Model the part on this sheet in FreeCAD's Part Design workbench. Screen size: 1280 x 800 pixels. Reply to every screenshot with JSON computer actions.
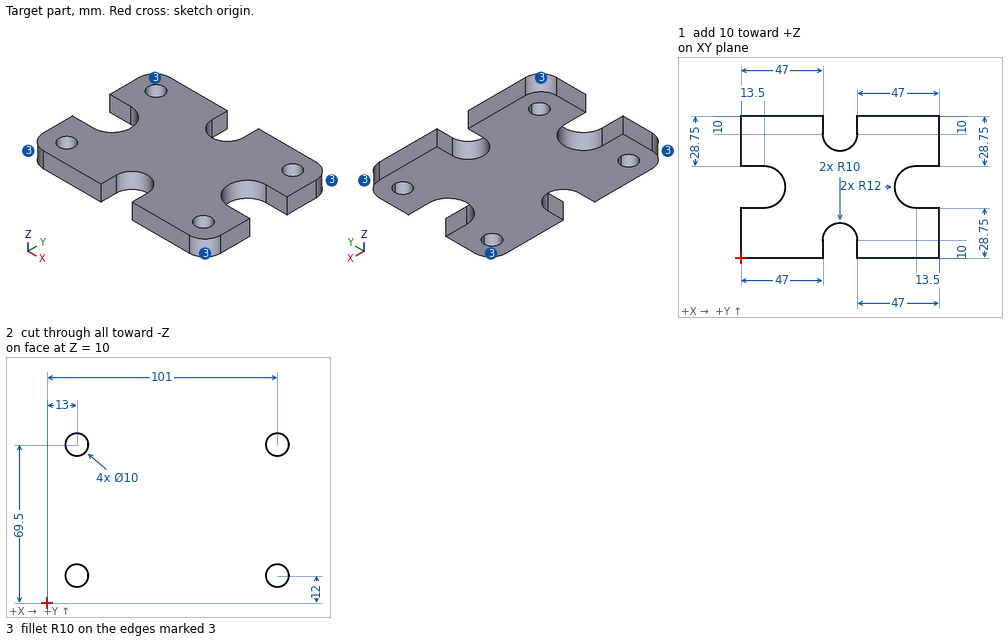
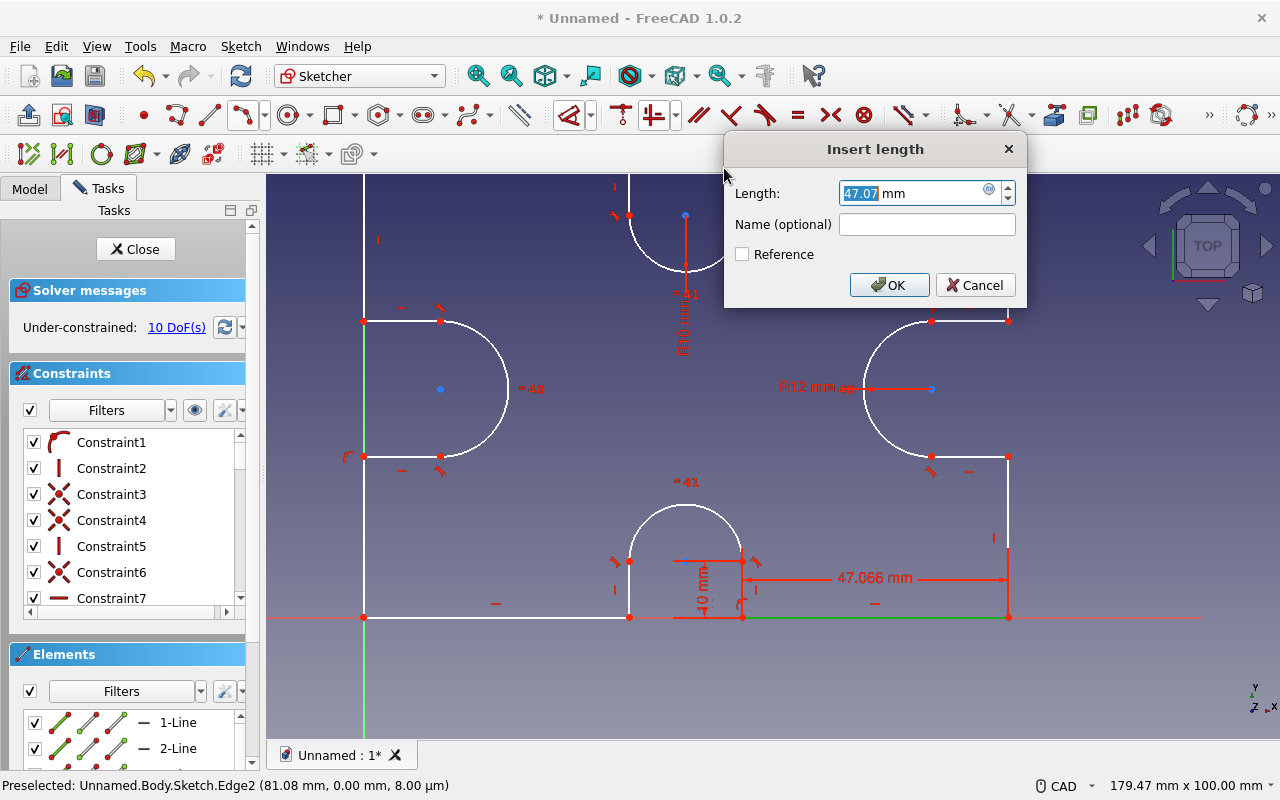
{"action": "type", "text": "47"}
{"action": "key", "text": "Return"}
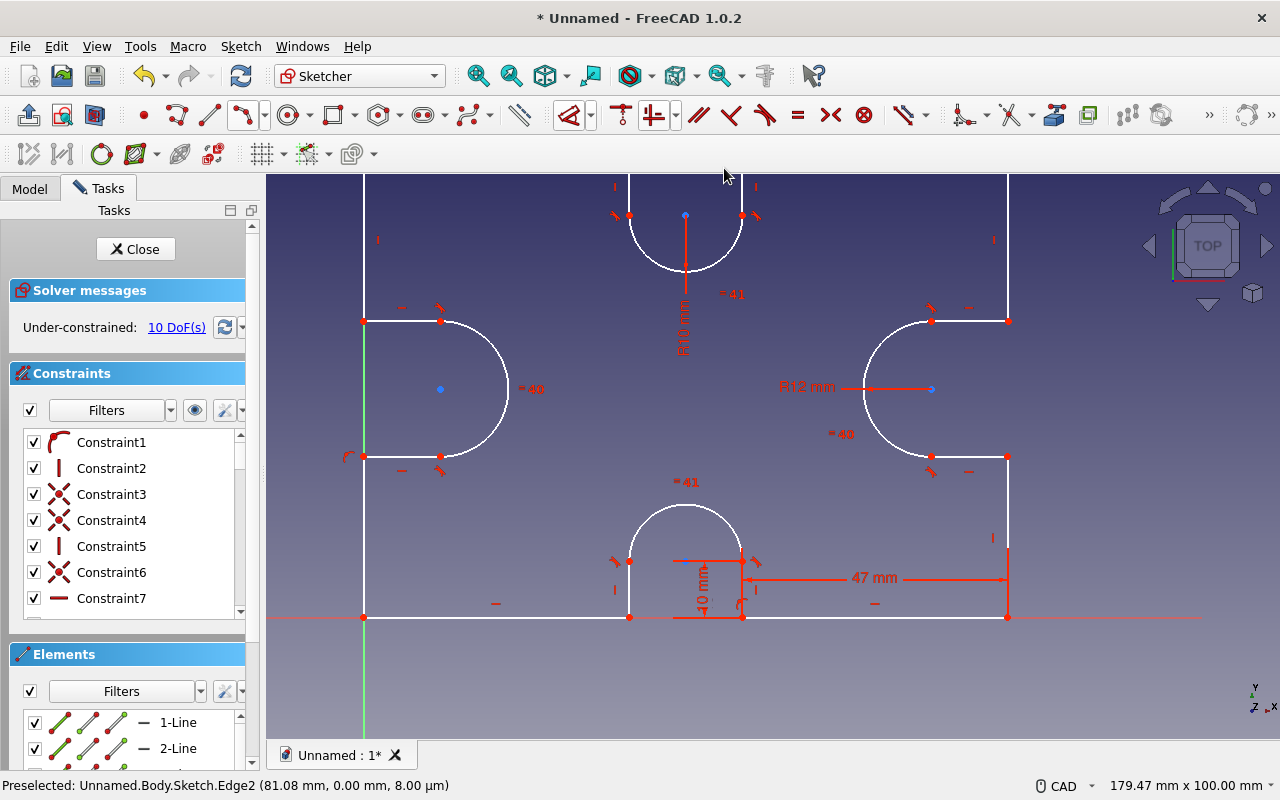
{"action": "scroll", "coordinate": [788, 711], "scroll_direction": "down", "scroll_amount": 1}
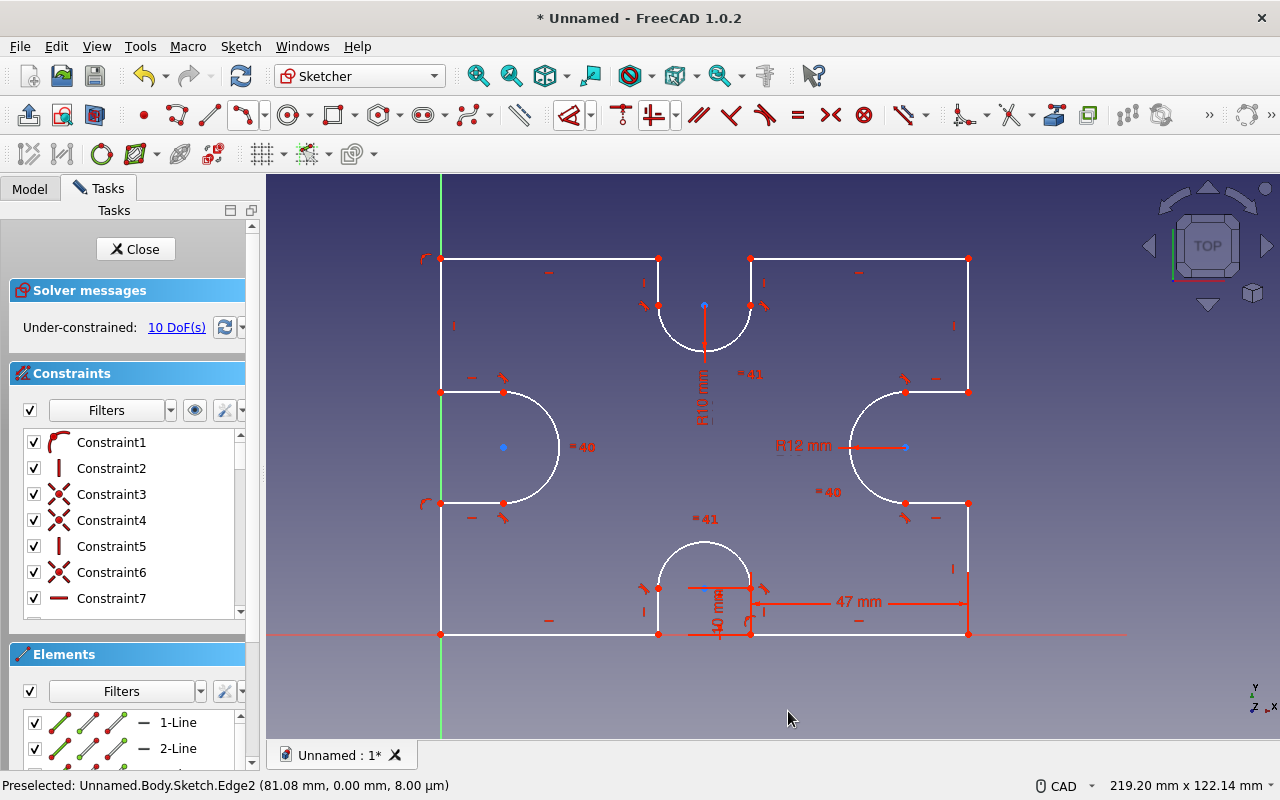
{"action": "left_click", "coordinate": [903, 259]}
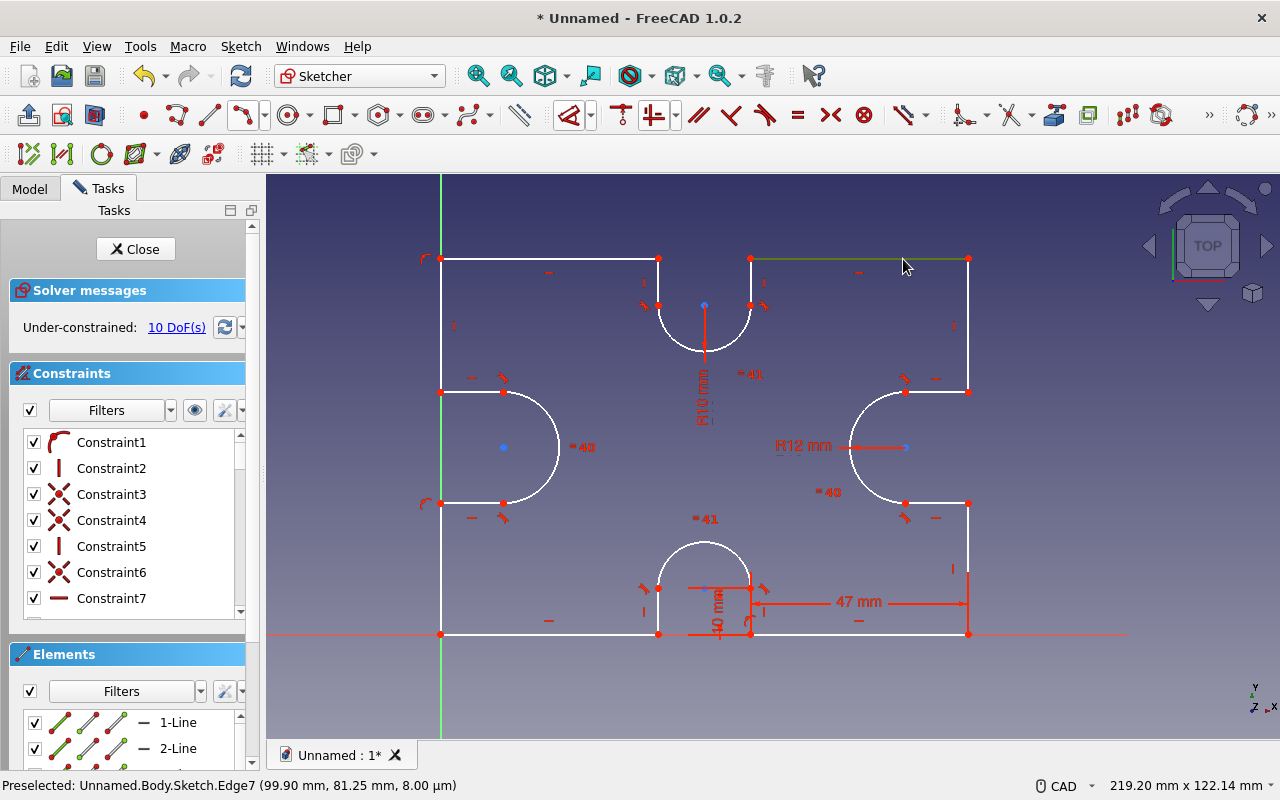
{"action": "left_click", "coordinate": [590, 116]}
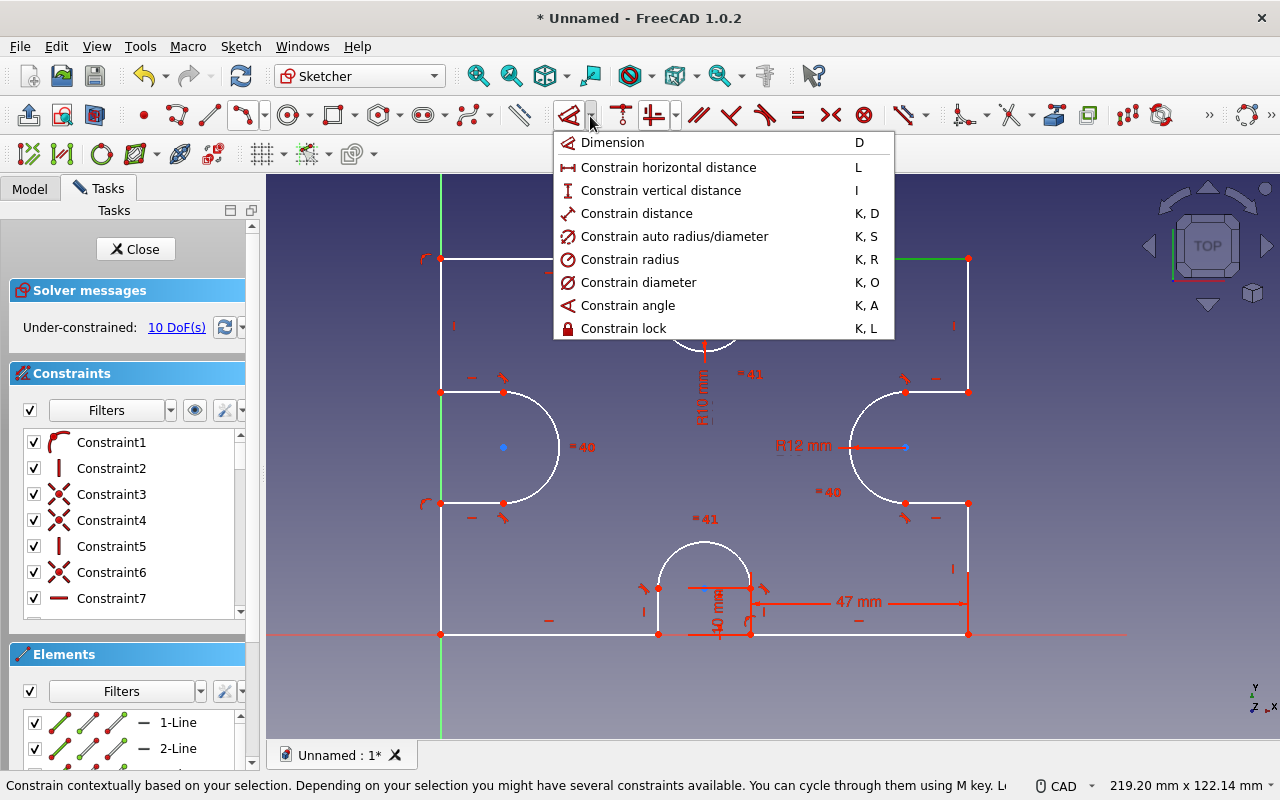
{"action": "left_click", "coordinate": [724, 168]}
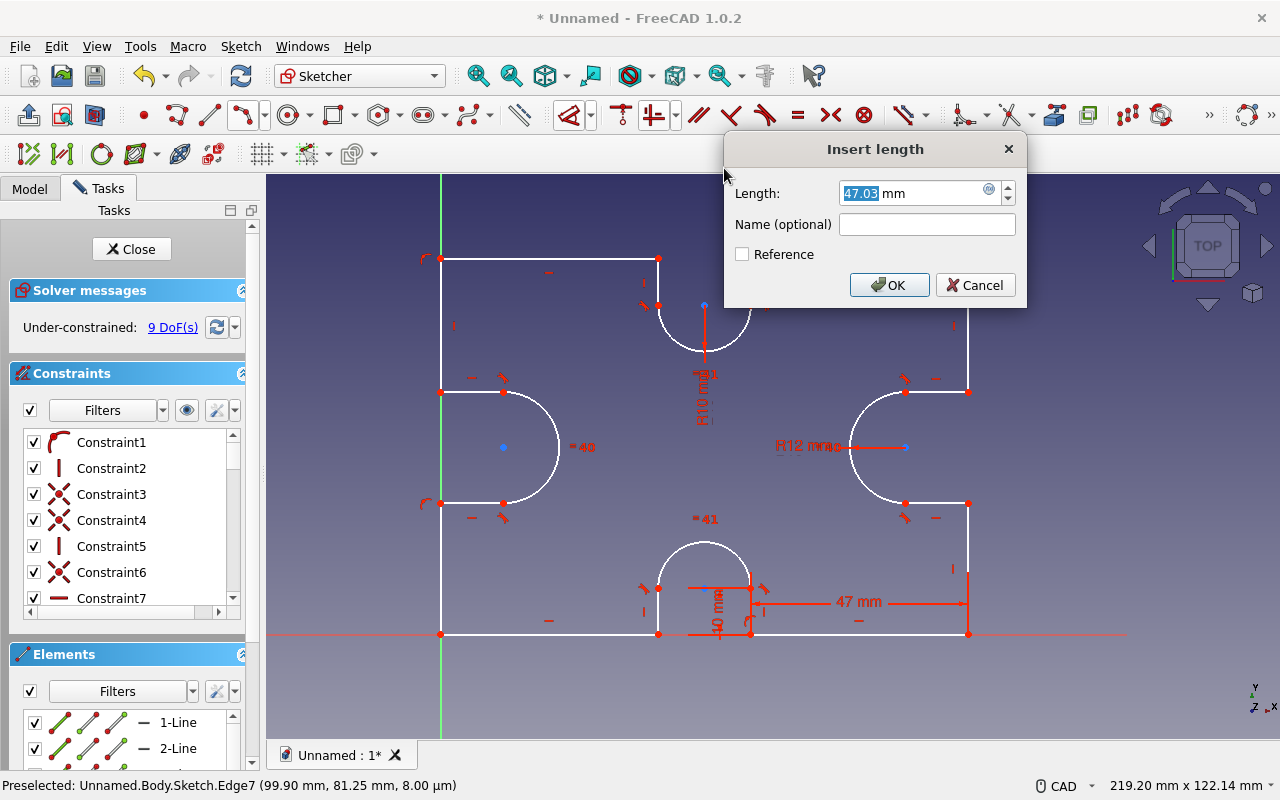
{"action": "type", "text": "47"}
{"action": "key", "text": "Return"}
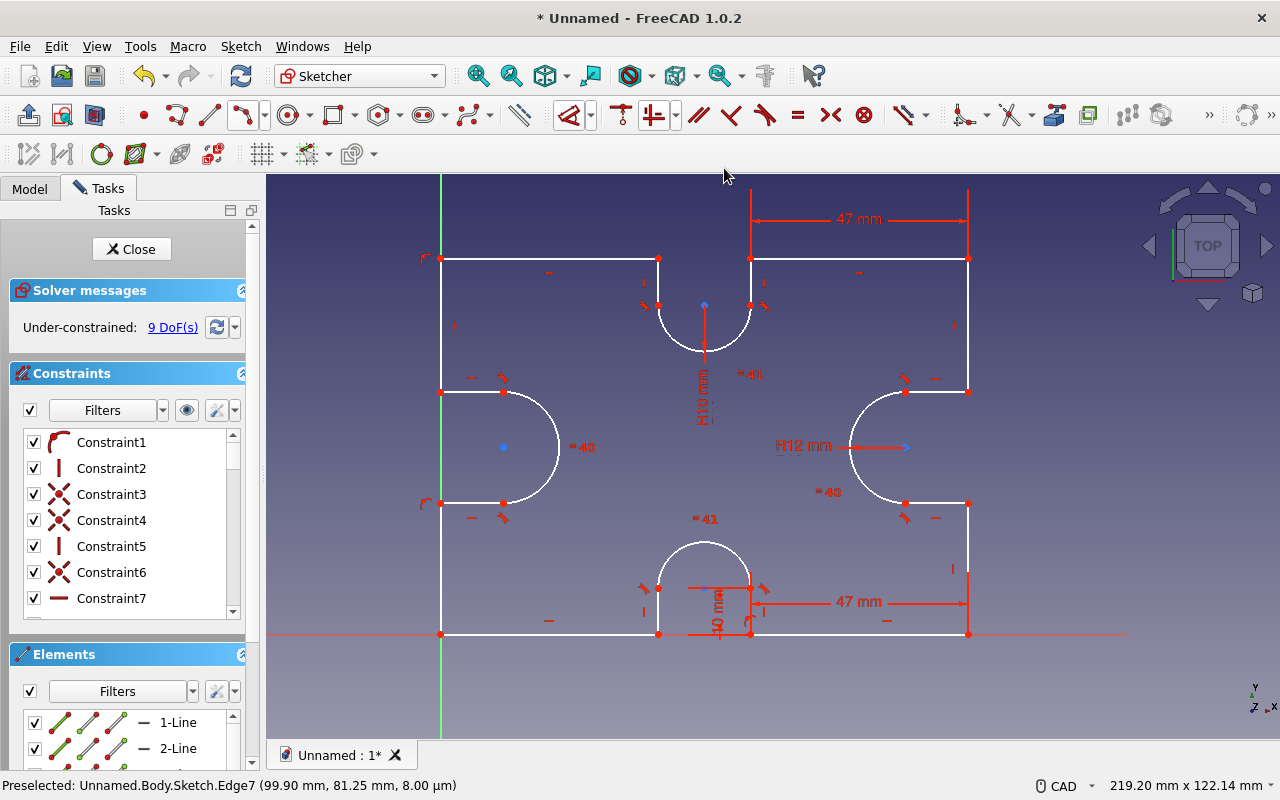
{"action": "left_click", "coordinate": [751, 273]}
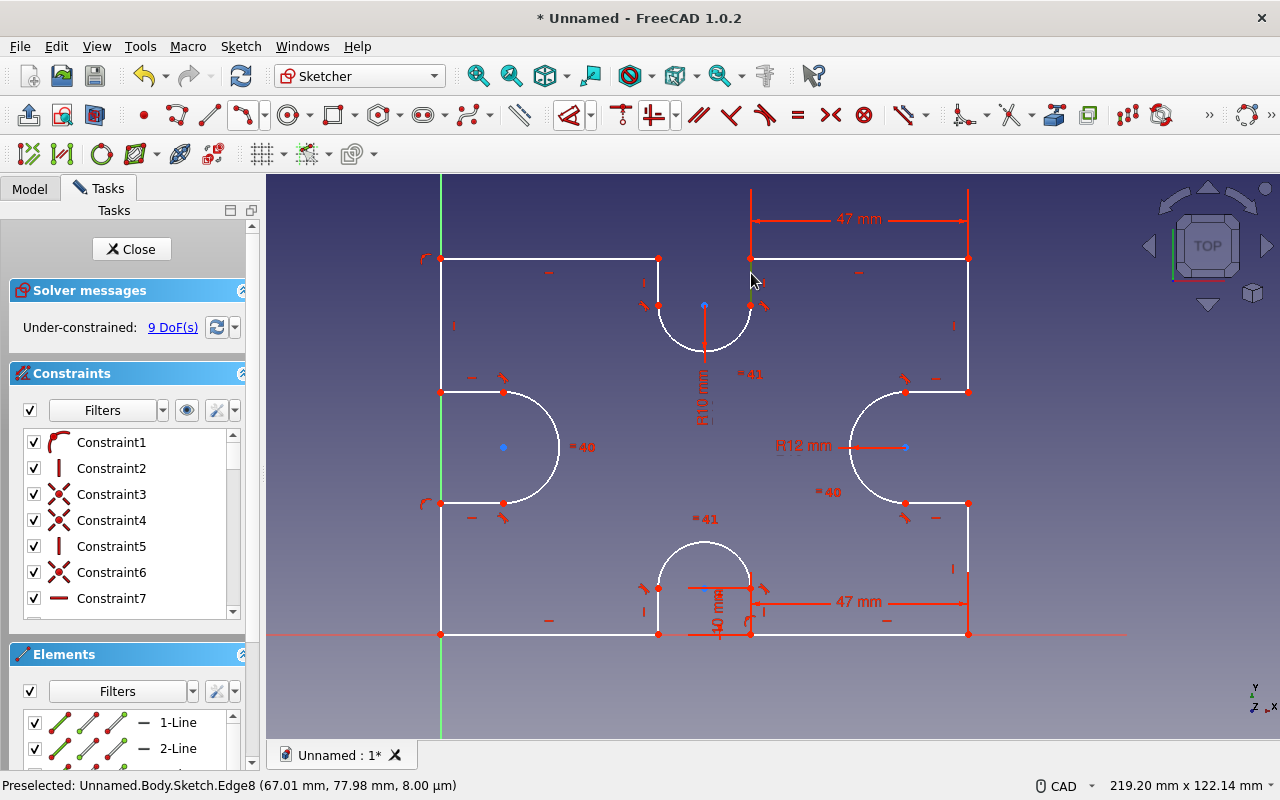
{"action": "left_click", "coordinate": [590, 116]}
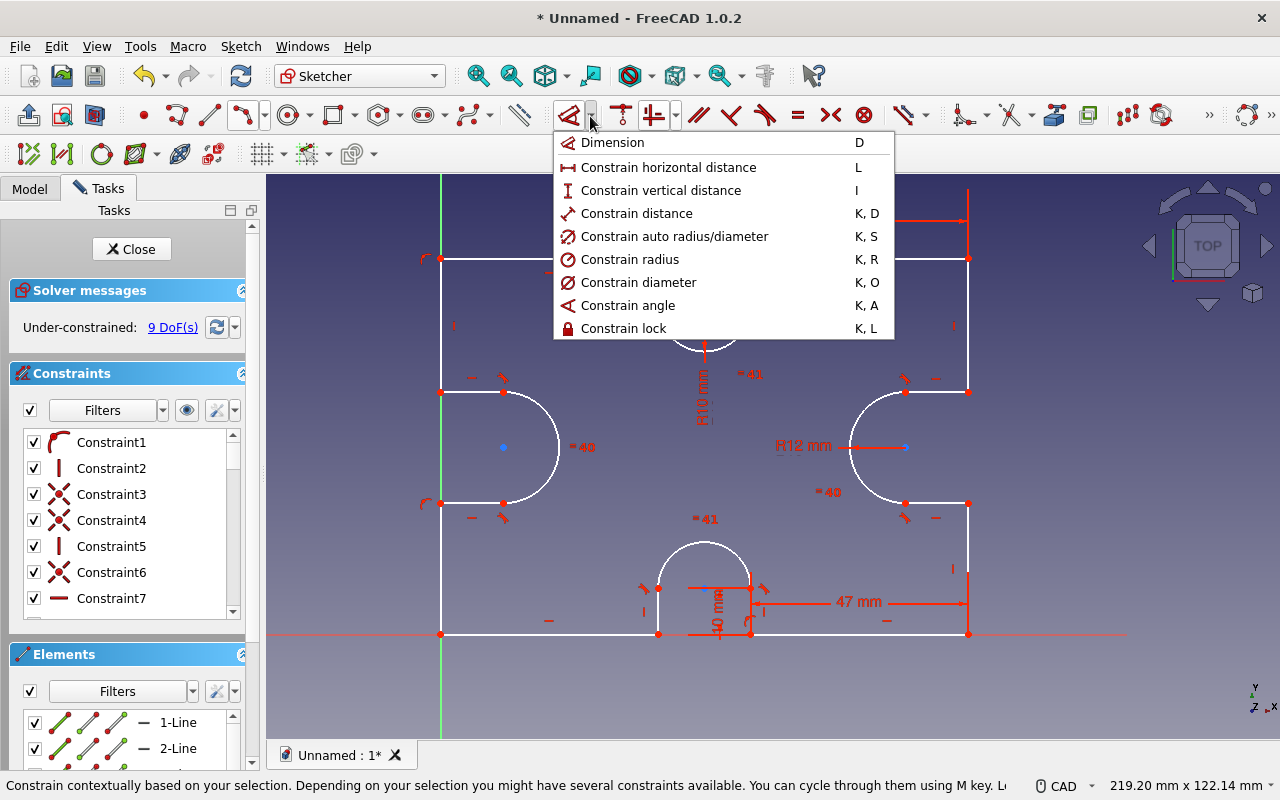
{"action": "left_click", "coordinate": [724, 190]}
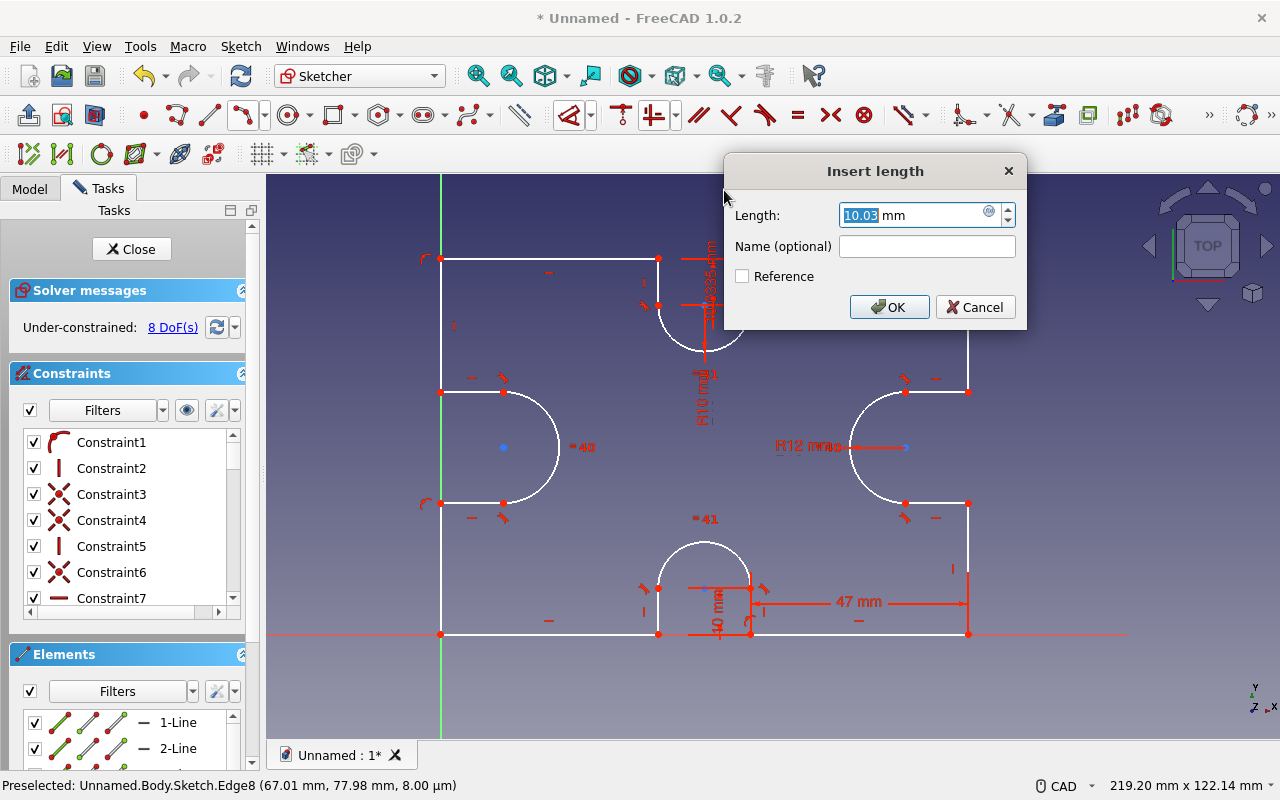
{"action": "type", "text": "10"}
{"action": "key", "text": "Return"}